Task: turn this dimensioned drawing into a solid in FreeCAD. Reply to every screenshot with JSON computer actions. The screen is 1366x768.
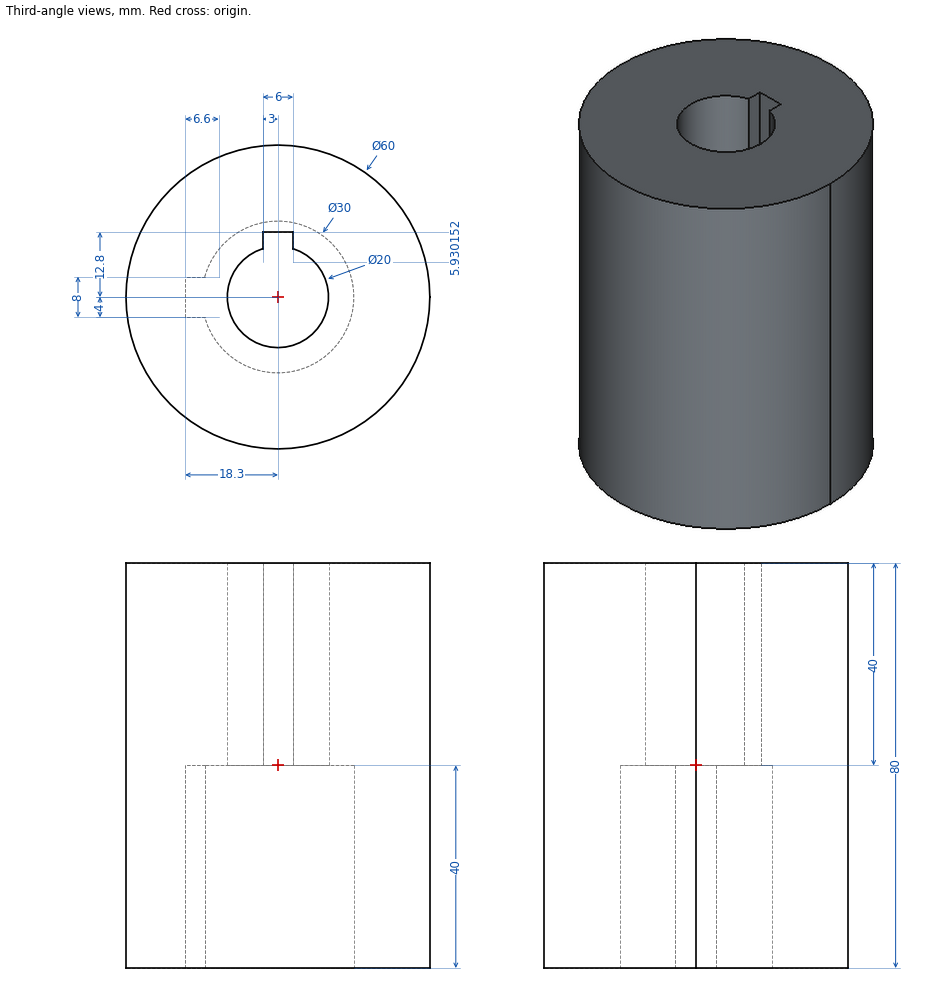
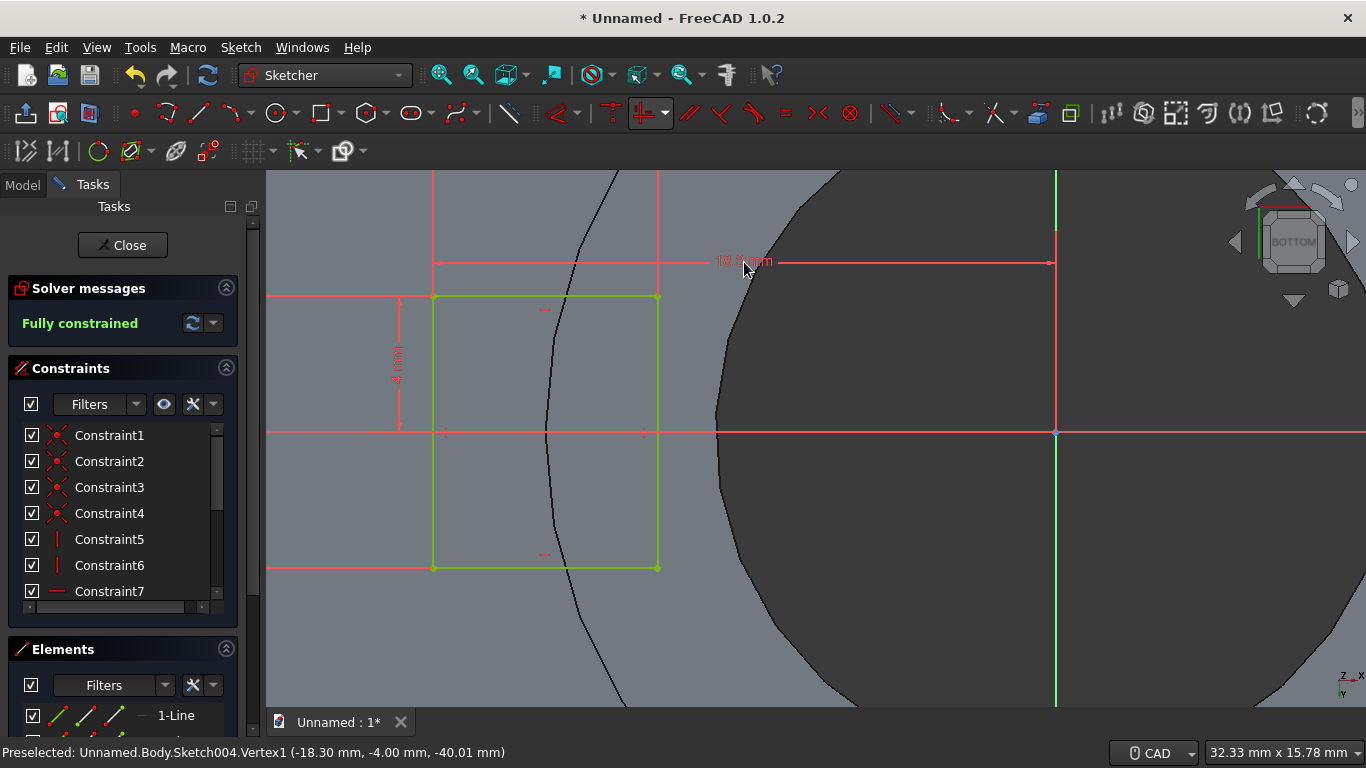
{"action": "left_click", "coordinate": [123, 245]}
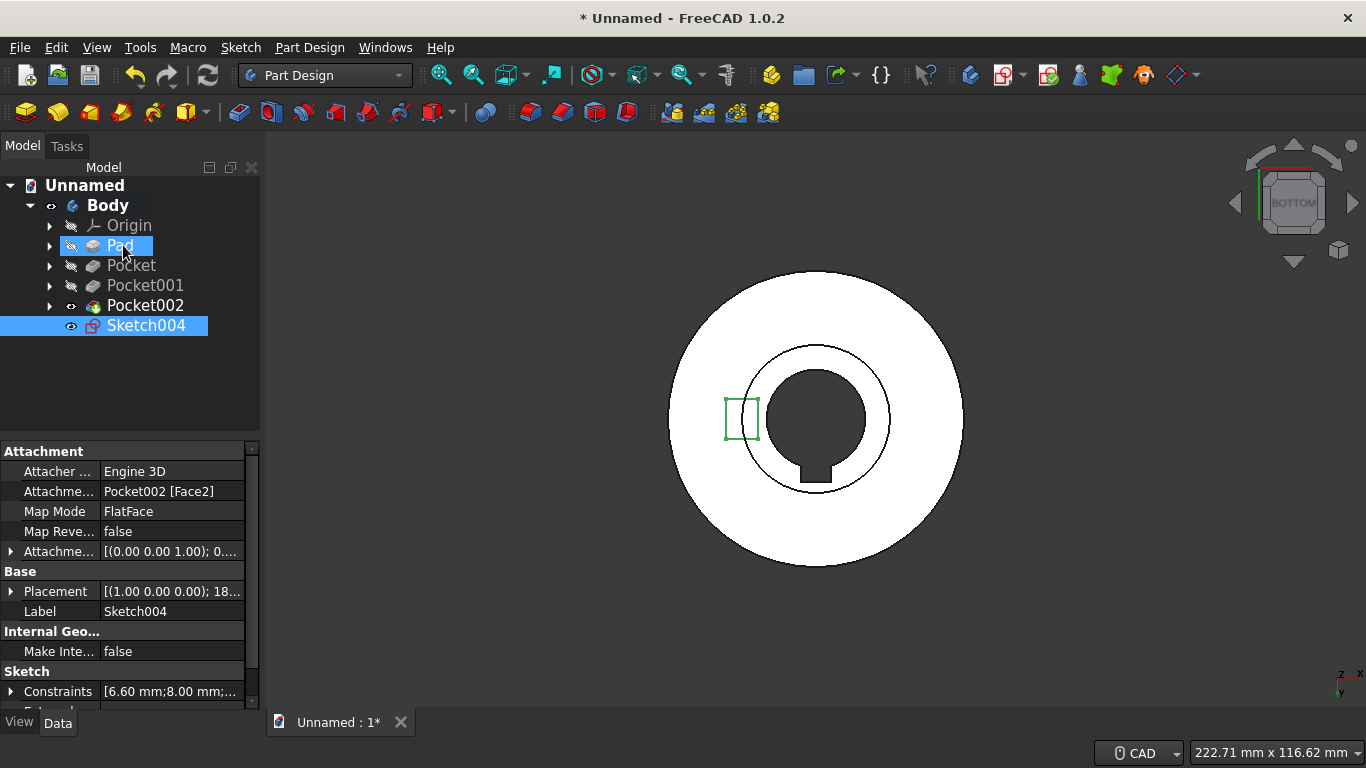
{"action": "left_click", "coordinate": [240, 112]}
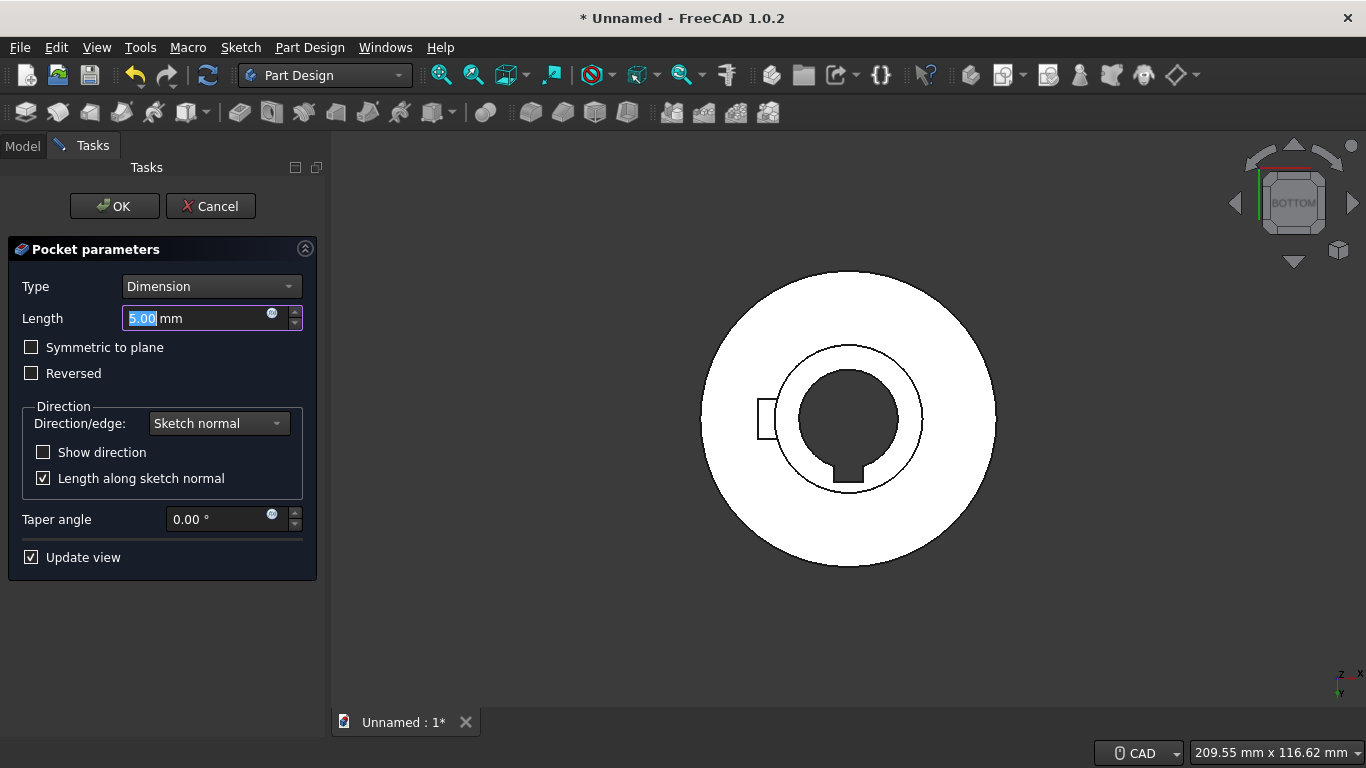
{"action": "type", "text": "40"}
{"action": "key", "text": "Tab"}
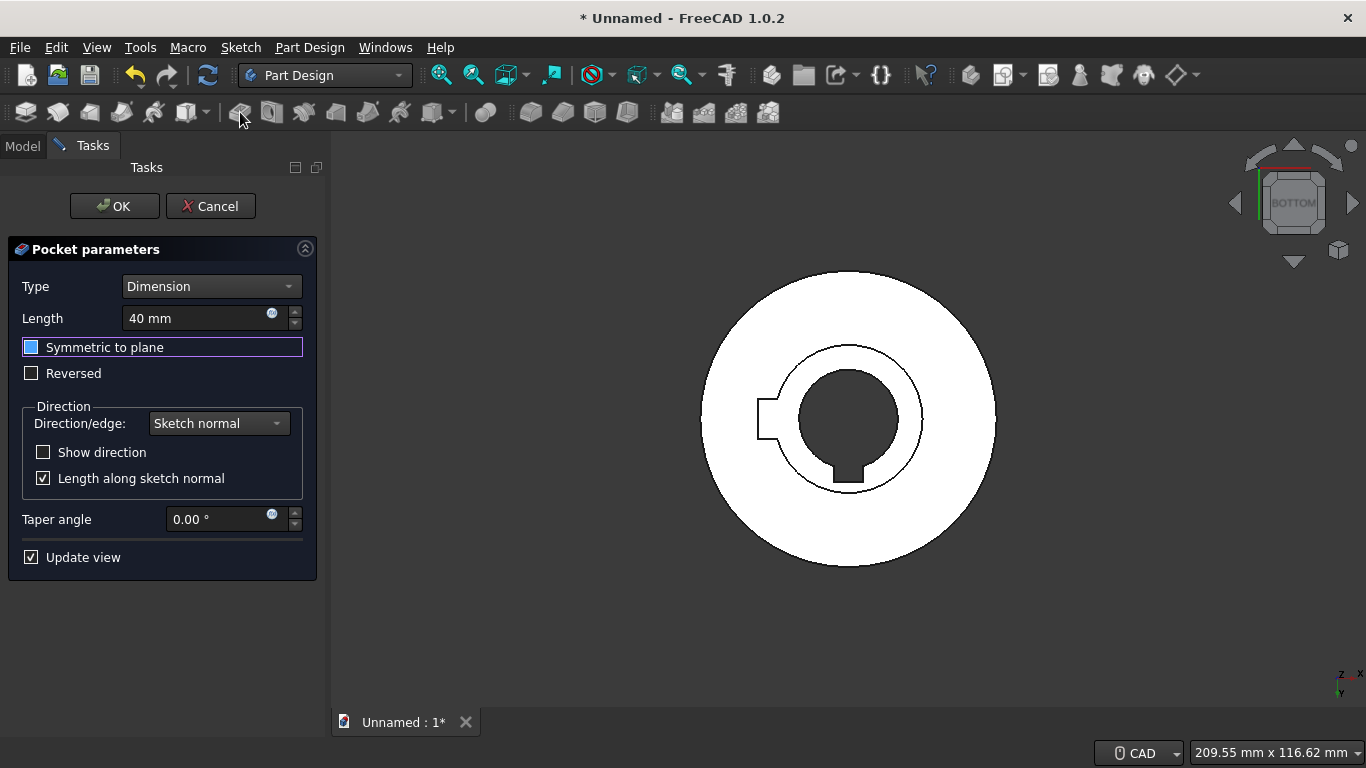
{"action": "left_click", "coordinate": [115, 206]}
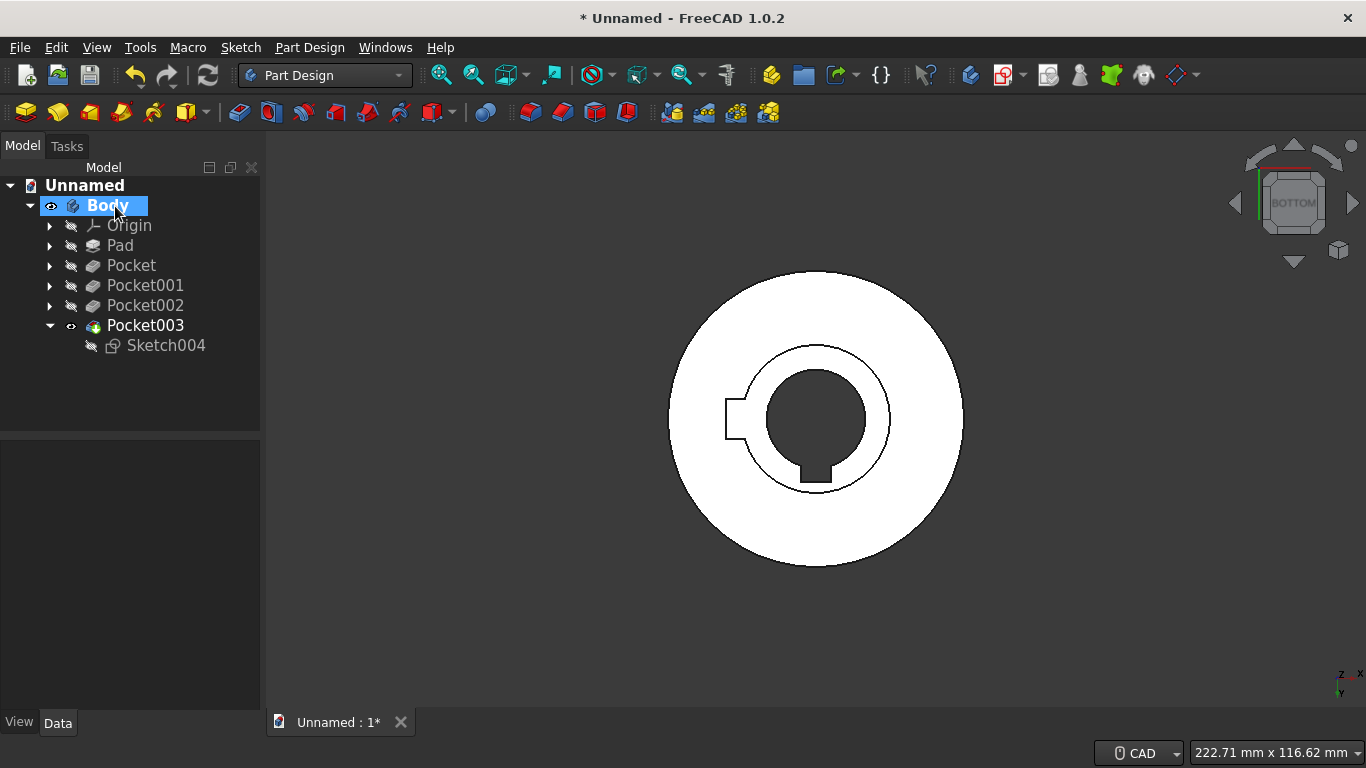
{"action": "key", "text": "0"}